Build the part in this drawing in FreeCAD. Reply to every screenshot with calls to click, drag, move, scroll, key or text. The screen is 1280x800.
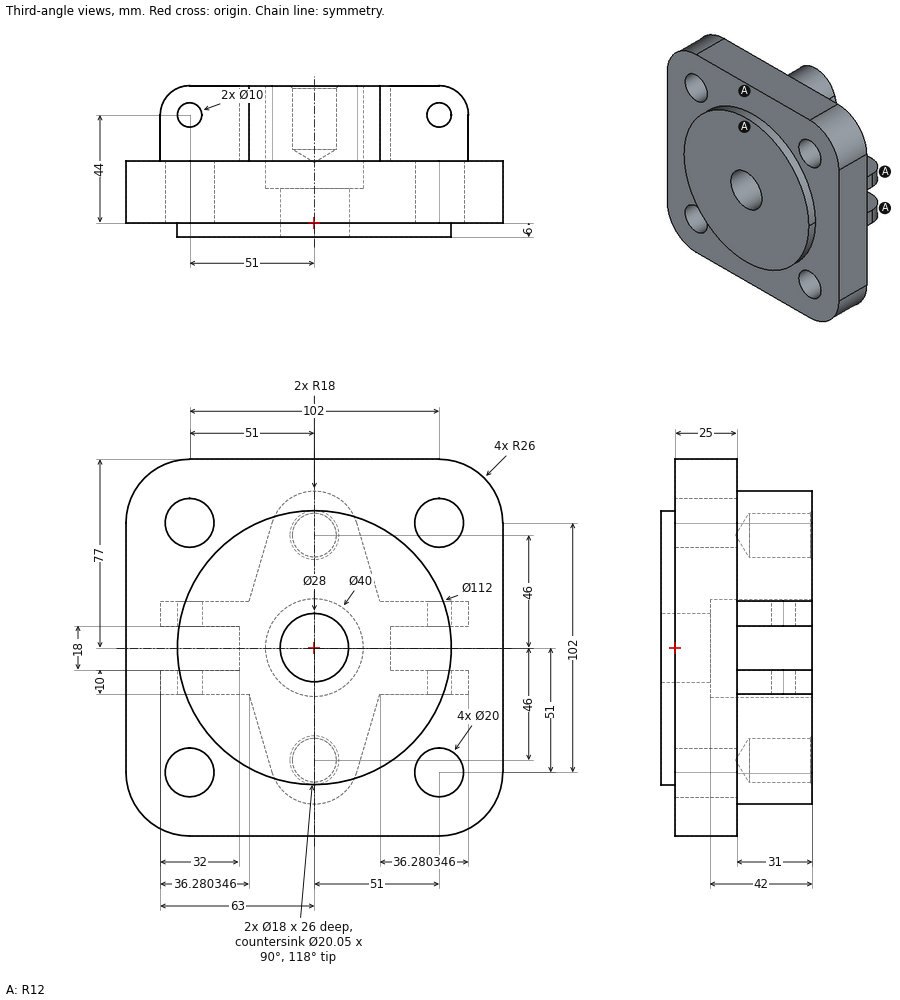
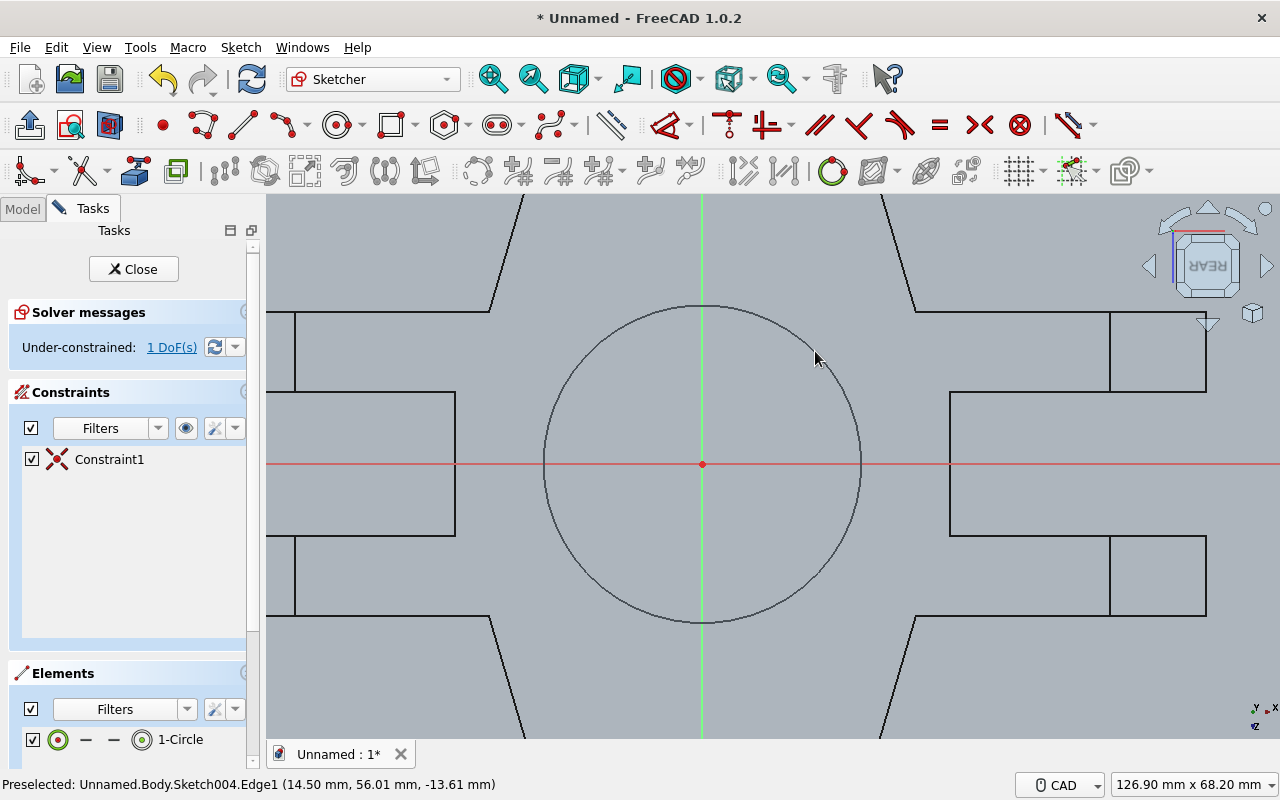
key(d)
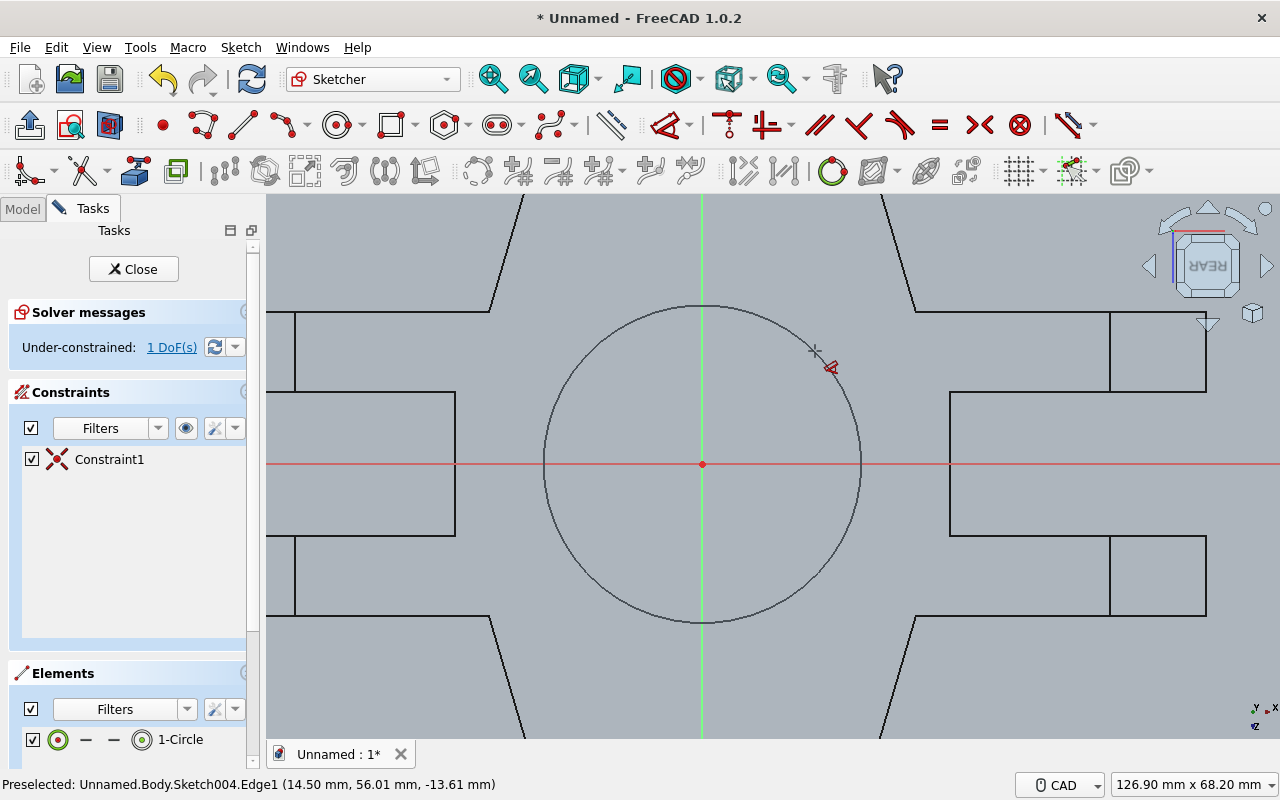
click(814, 351)
click(836, 328)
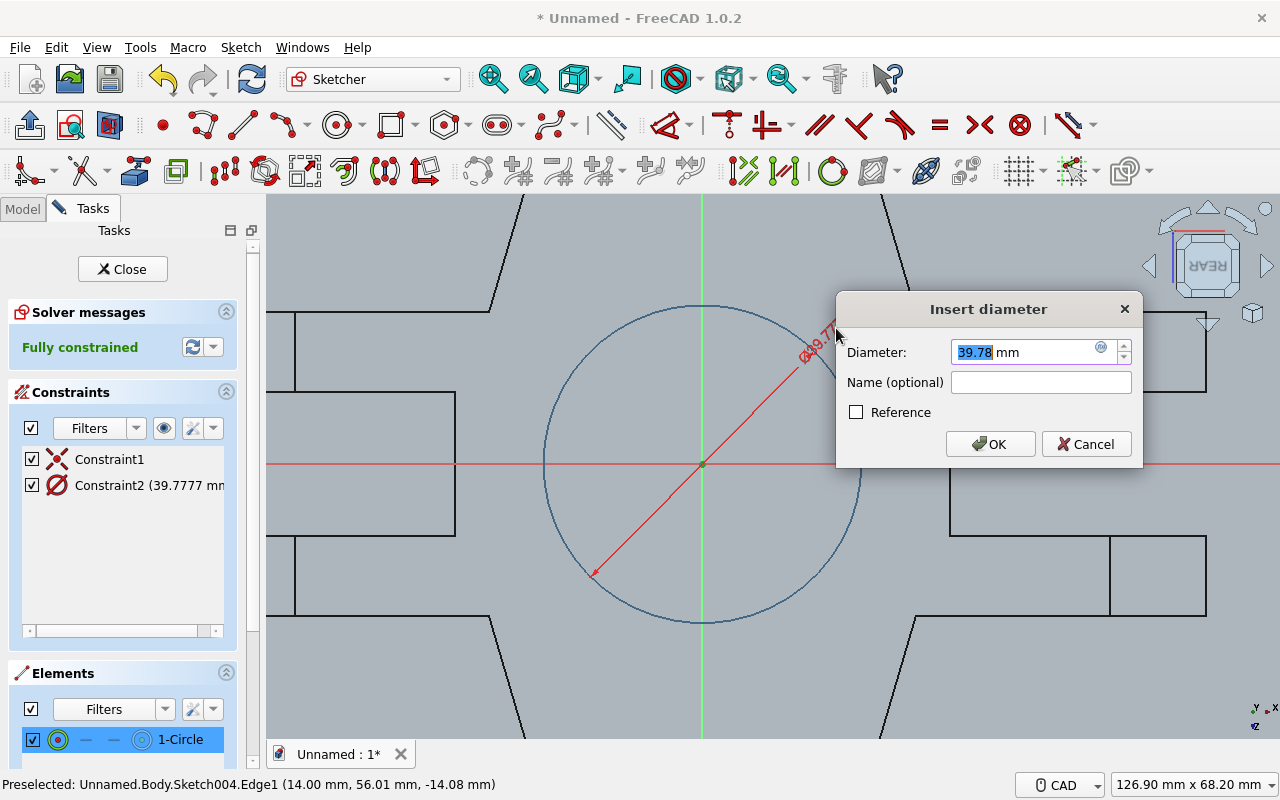
text(40)
key(Return)
key(Escape)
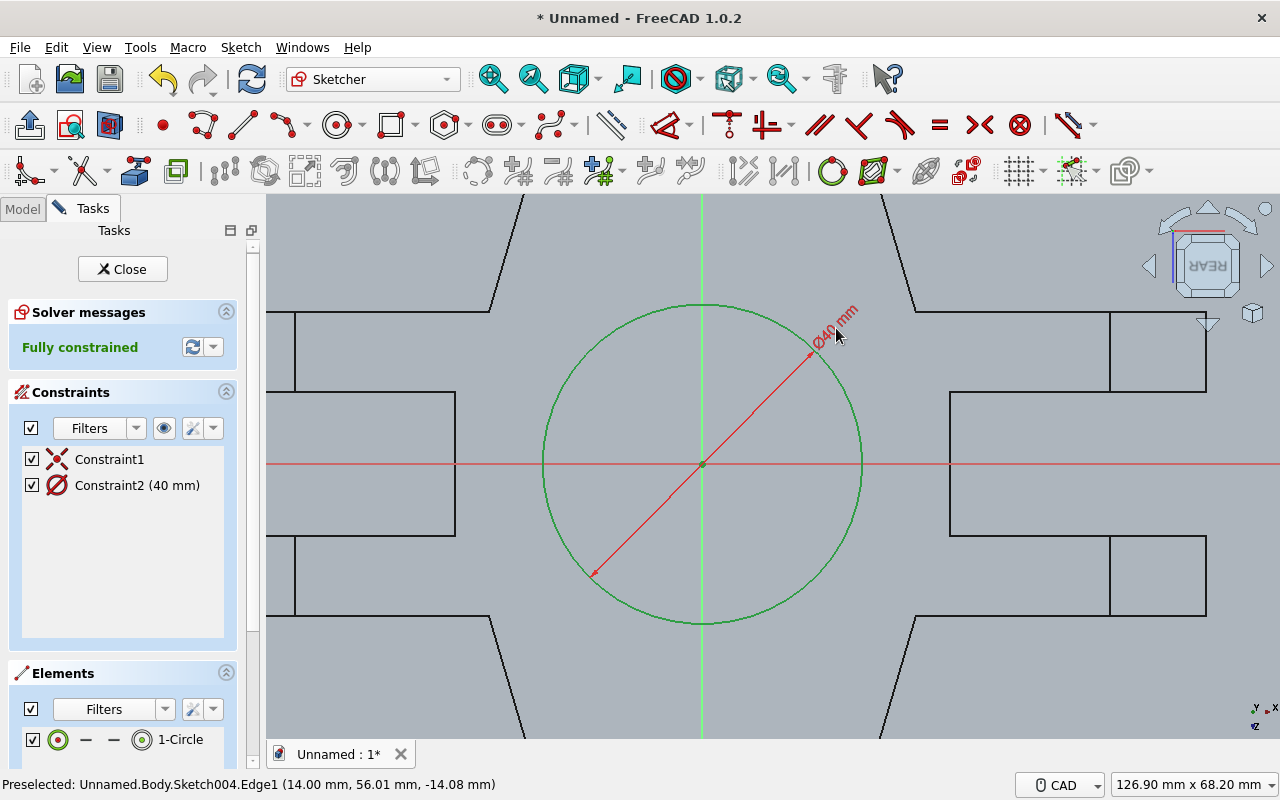
click(123, 269)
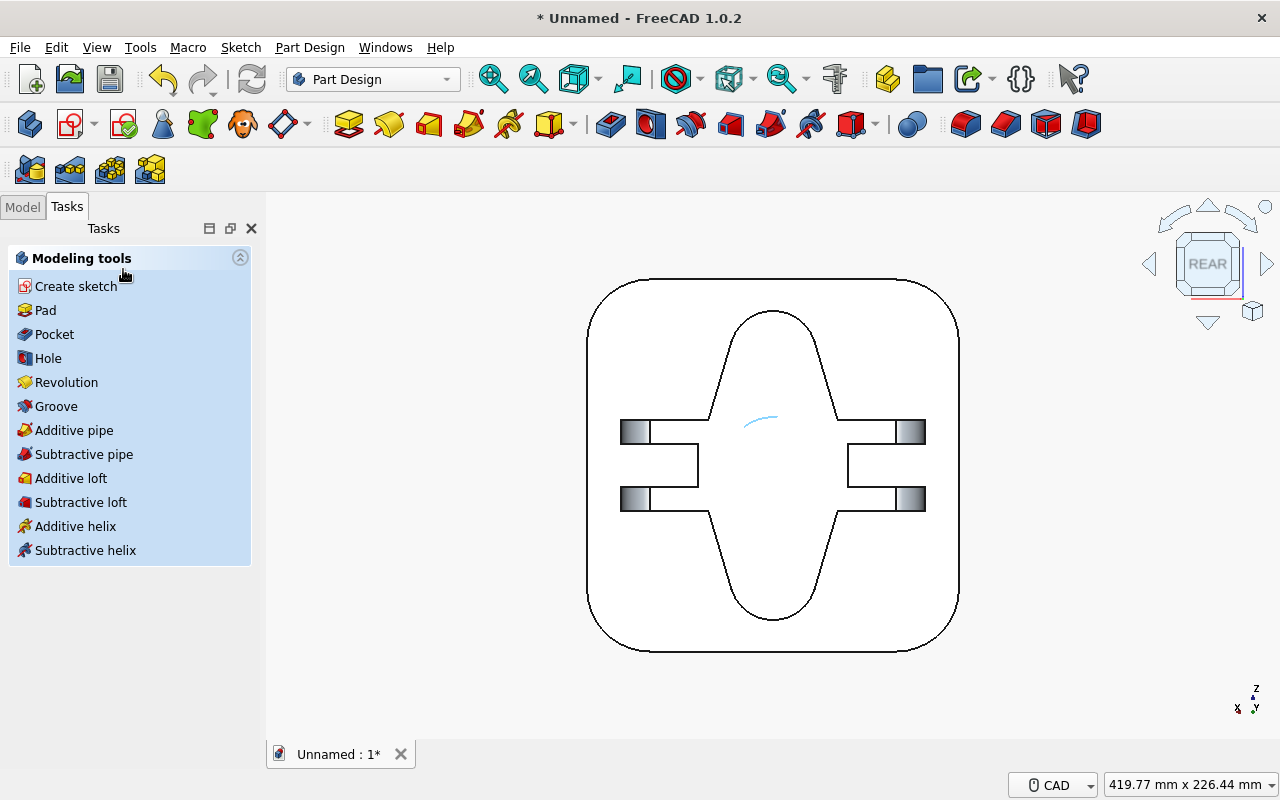
click(612, 124)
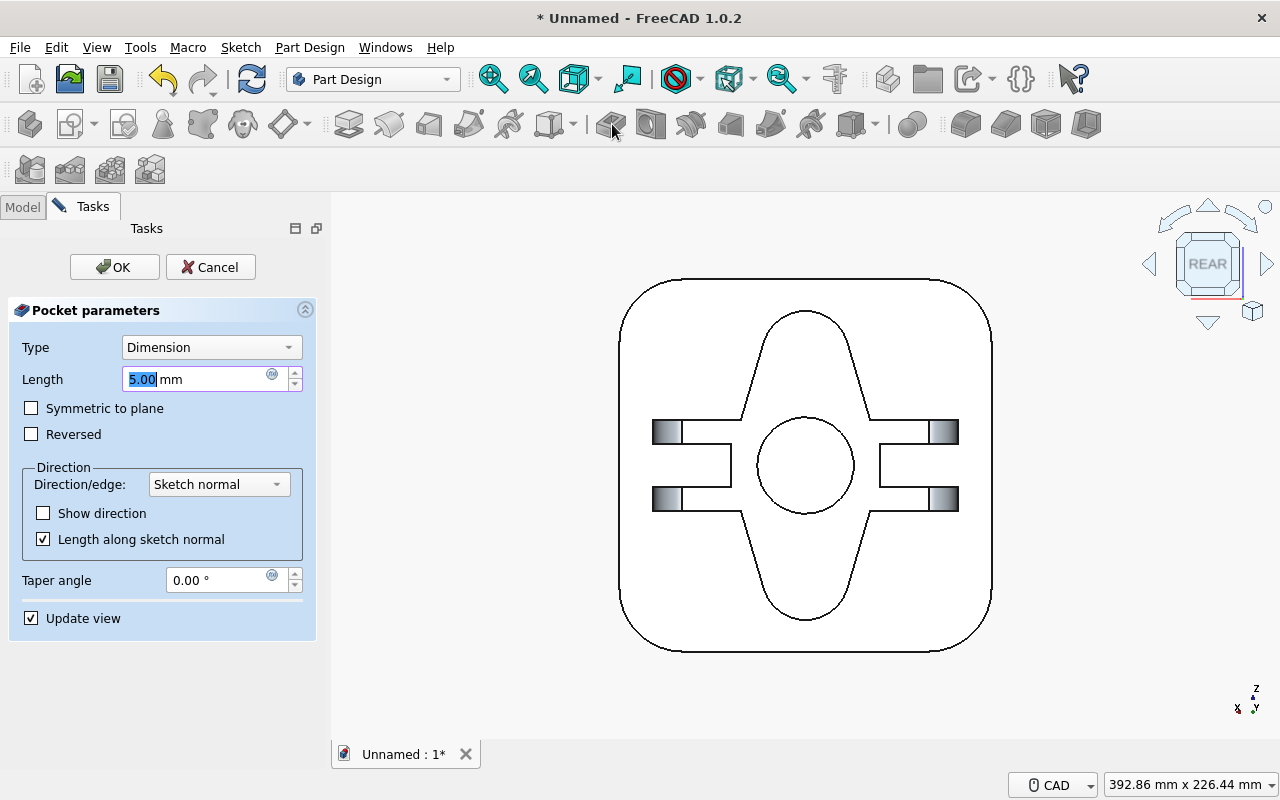
text(42)
key(Tab)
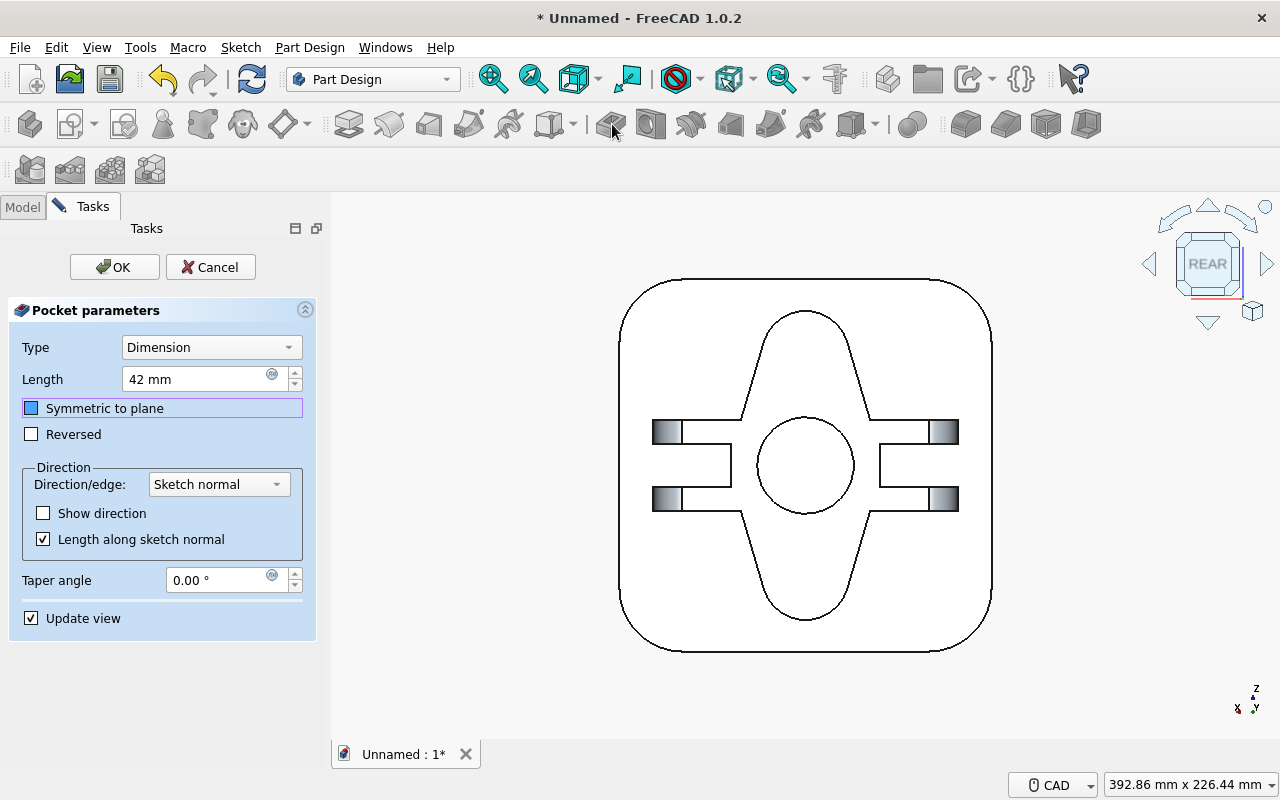
click(115, 267)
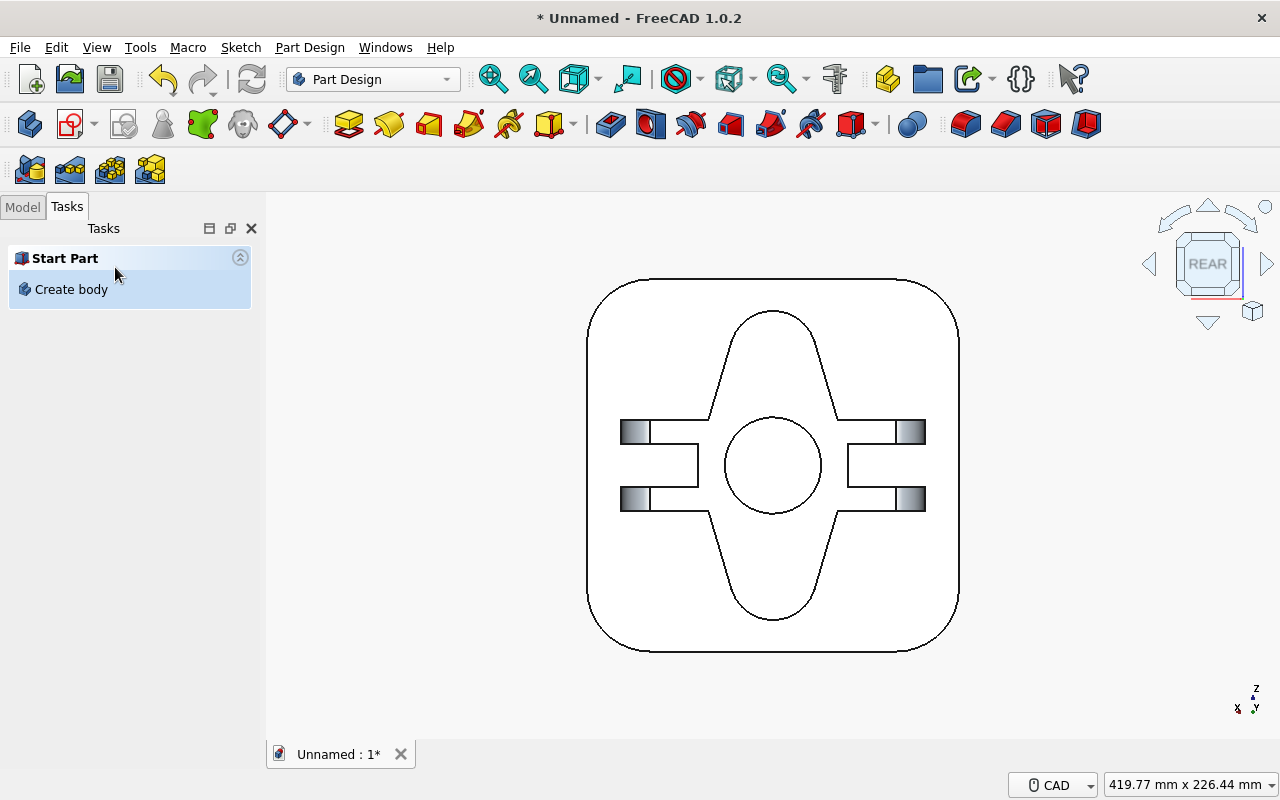
click(773, 464)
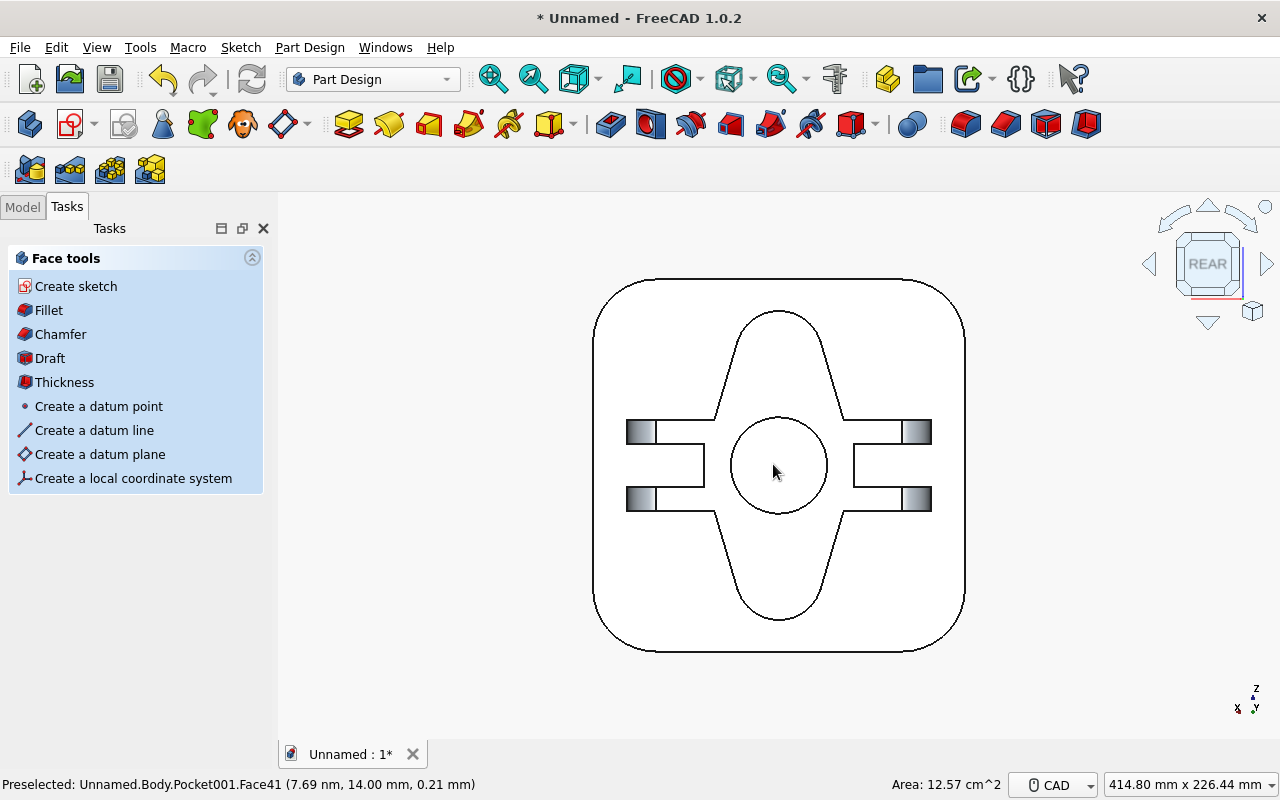
click(70, 124)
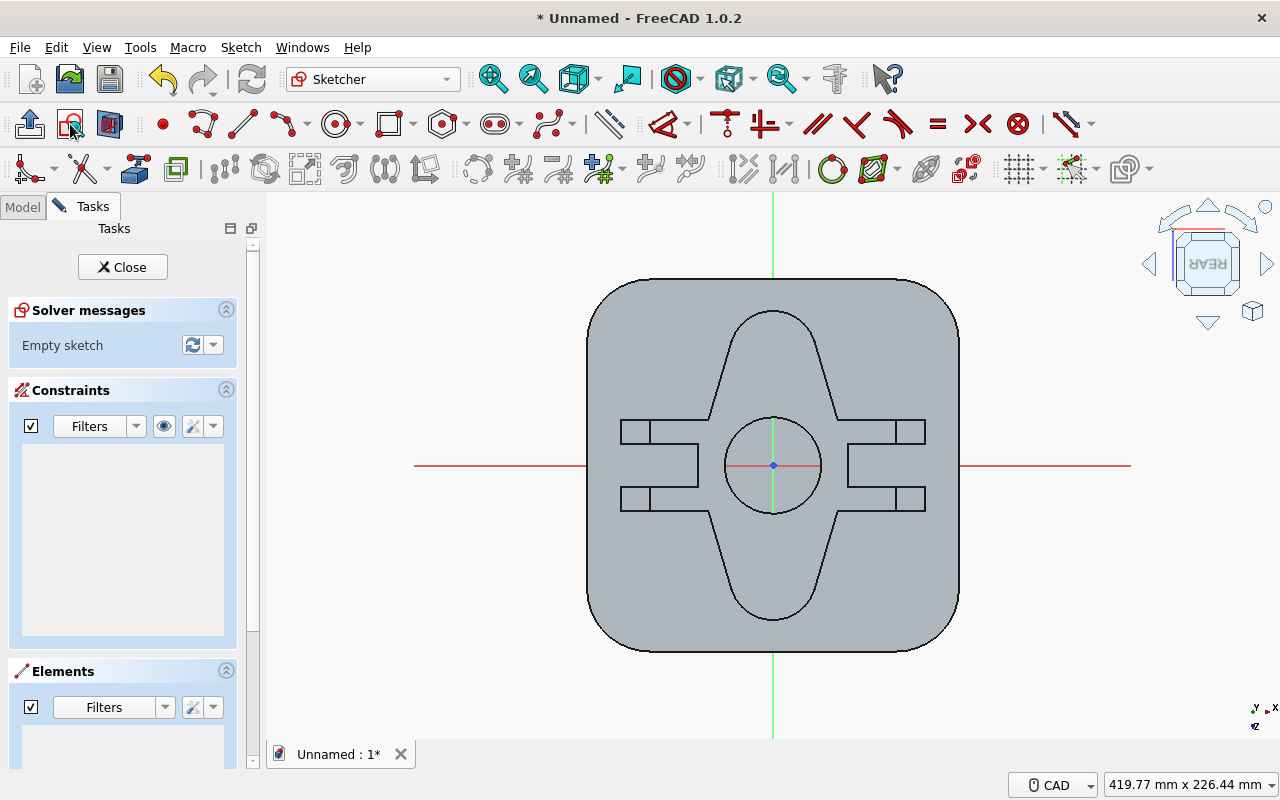
scroll(790, 465, up, 8)